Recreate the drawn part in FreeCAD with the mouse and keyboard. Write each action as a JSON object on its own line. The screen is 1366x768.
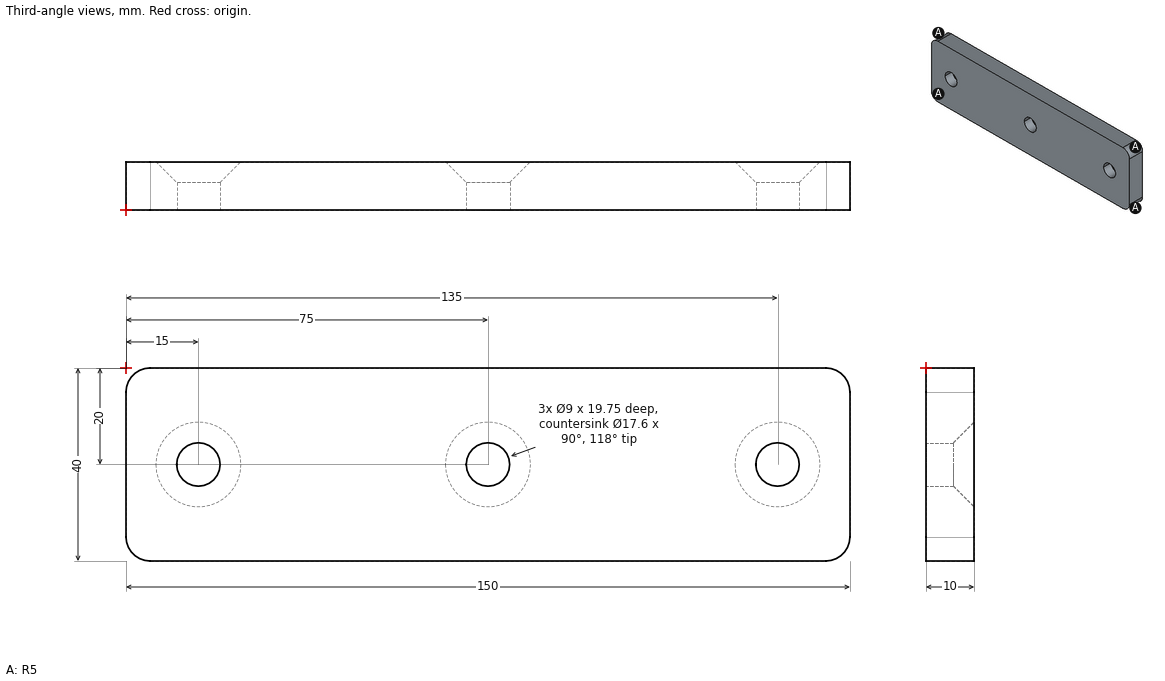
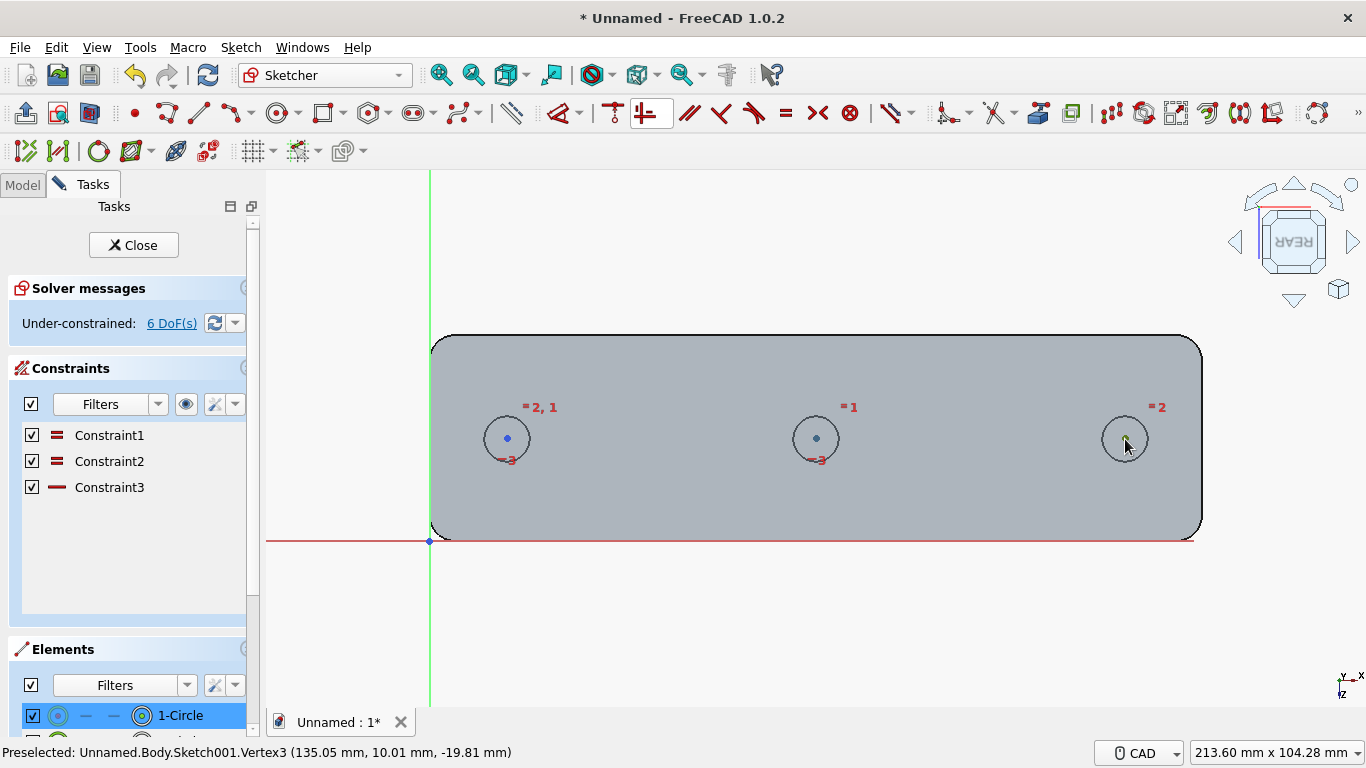
{"action": "left_click", "coordinate": [668, 114]}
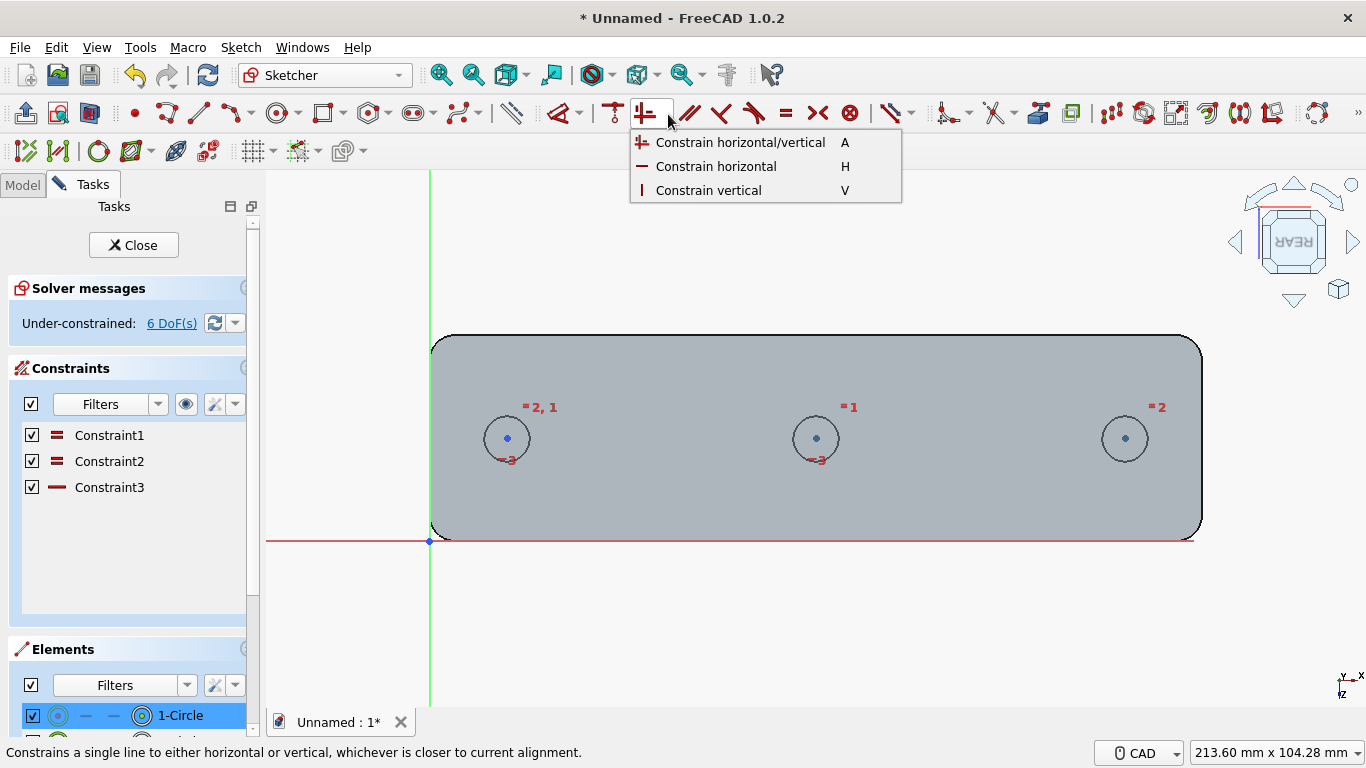
{"action": "left_click", "coordinate": [766, 166]}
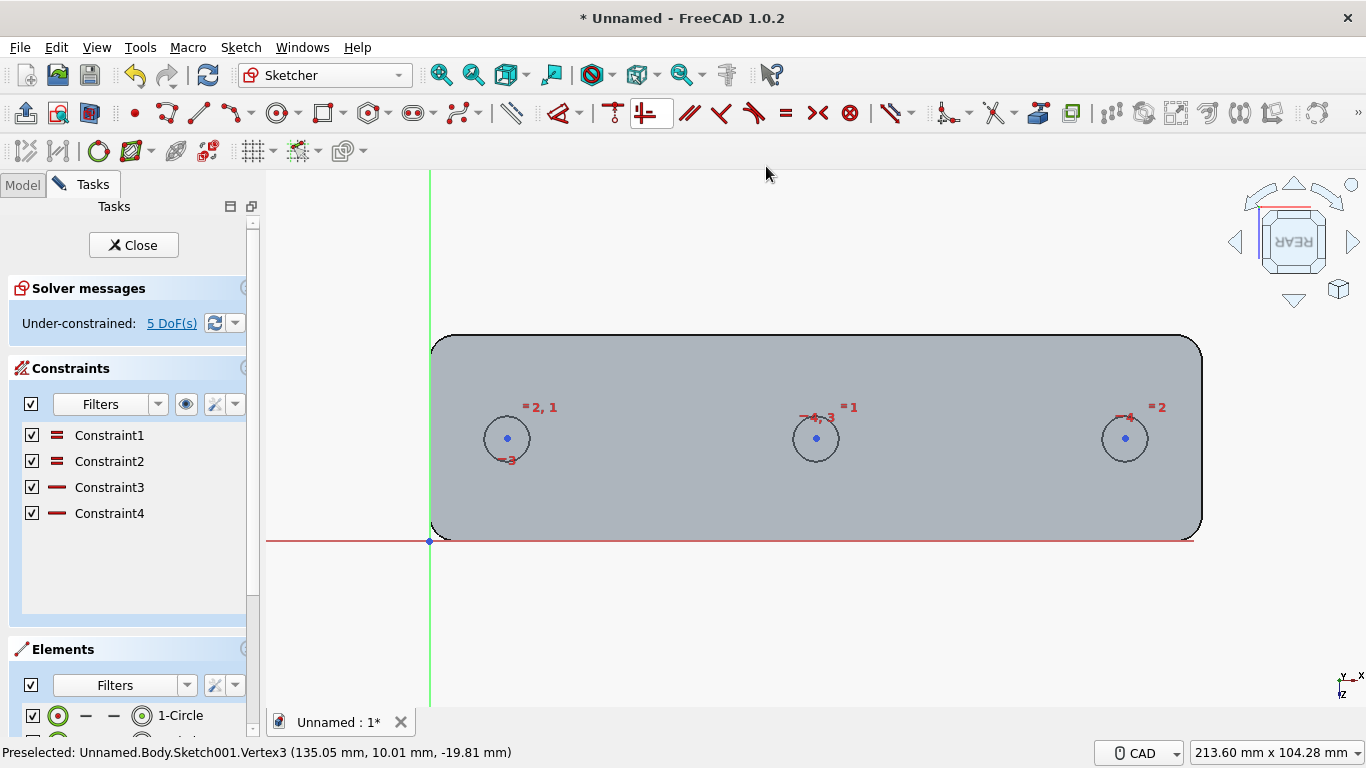
{"action": "left_click", "coordinate": [558, 114]}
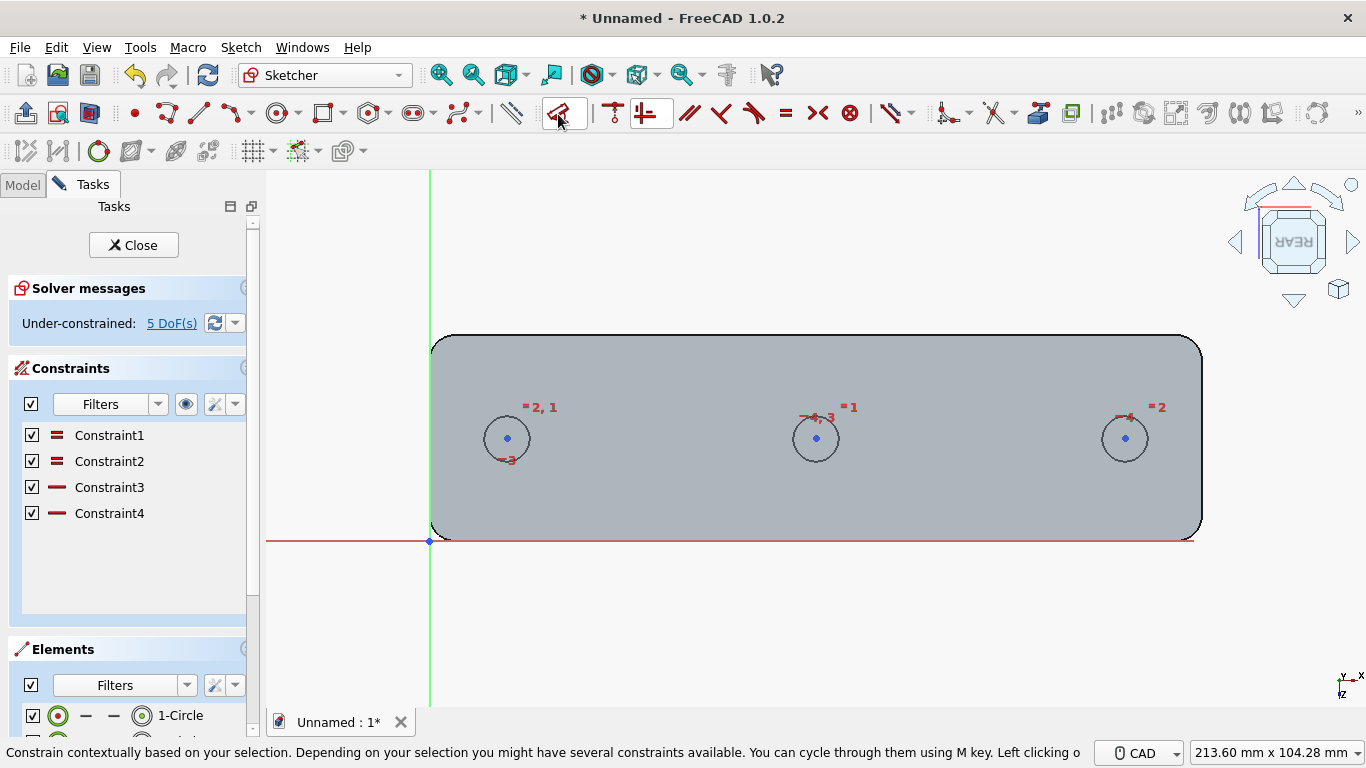
{"action": "left_click", "coordinate": [832, 423]}
{"action": "left_click", "coordinate": [855, 400]}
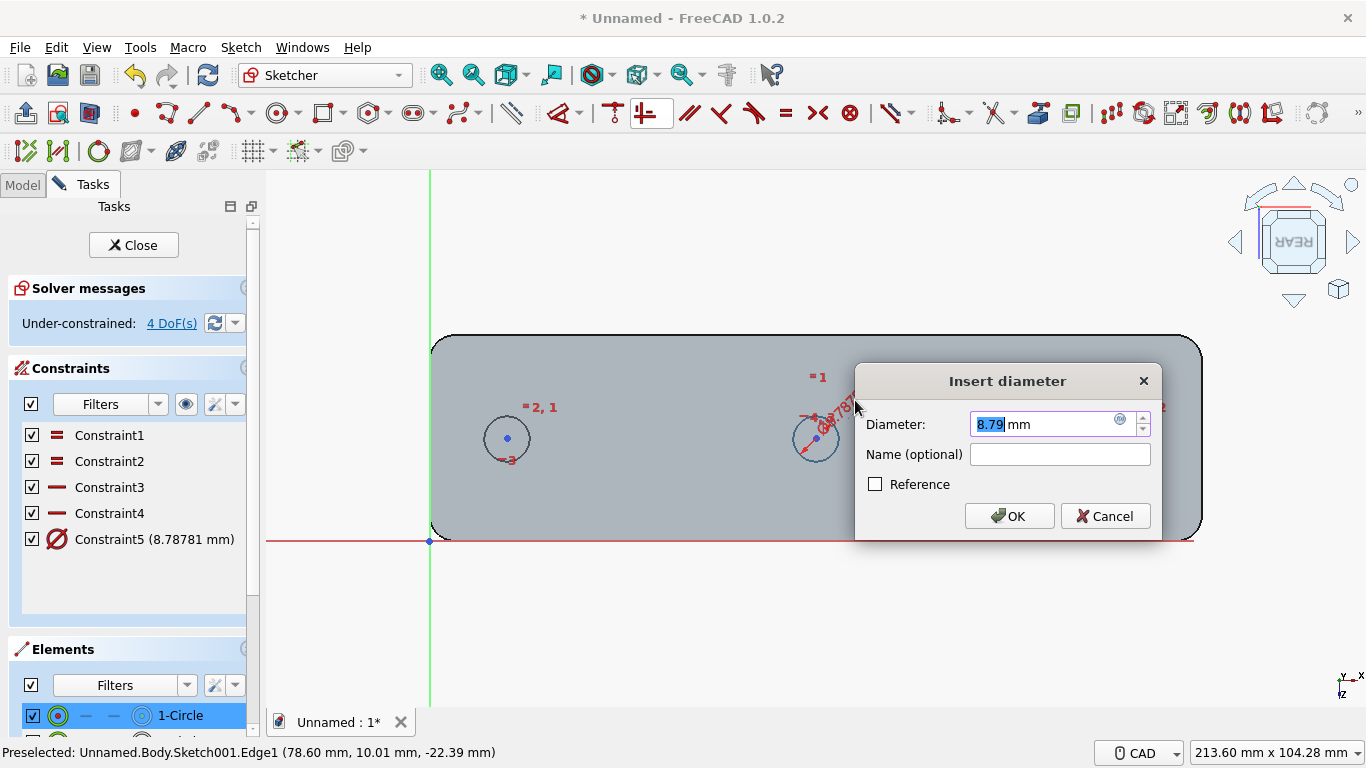
{"action": "type", "text": "9"}
{"action": "key", "text": "Return"}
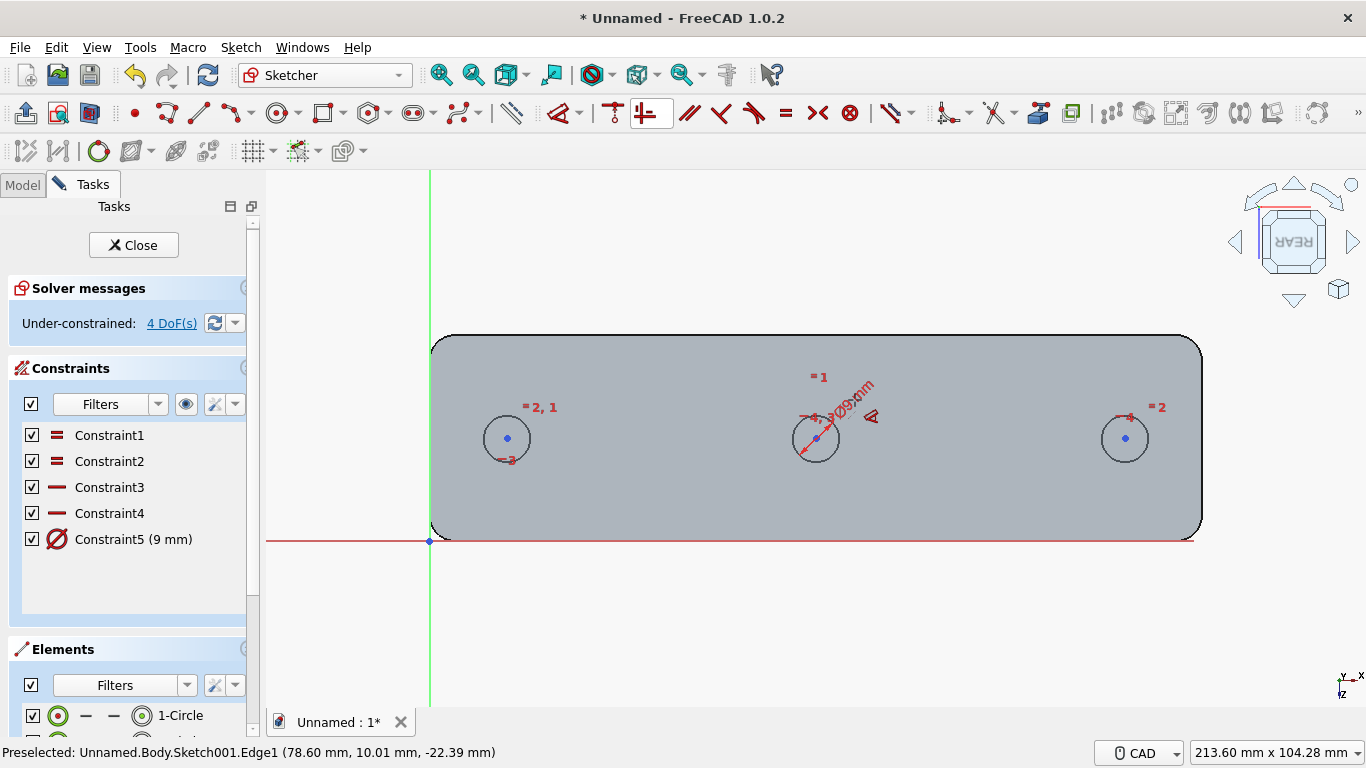
{"action": "left_click", "coordinate": [816, 439]}
{"action": "left_click", "coordinate": [623, 575]}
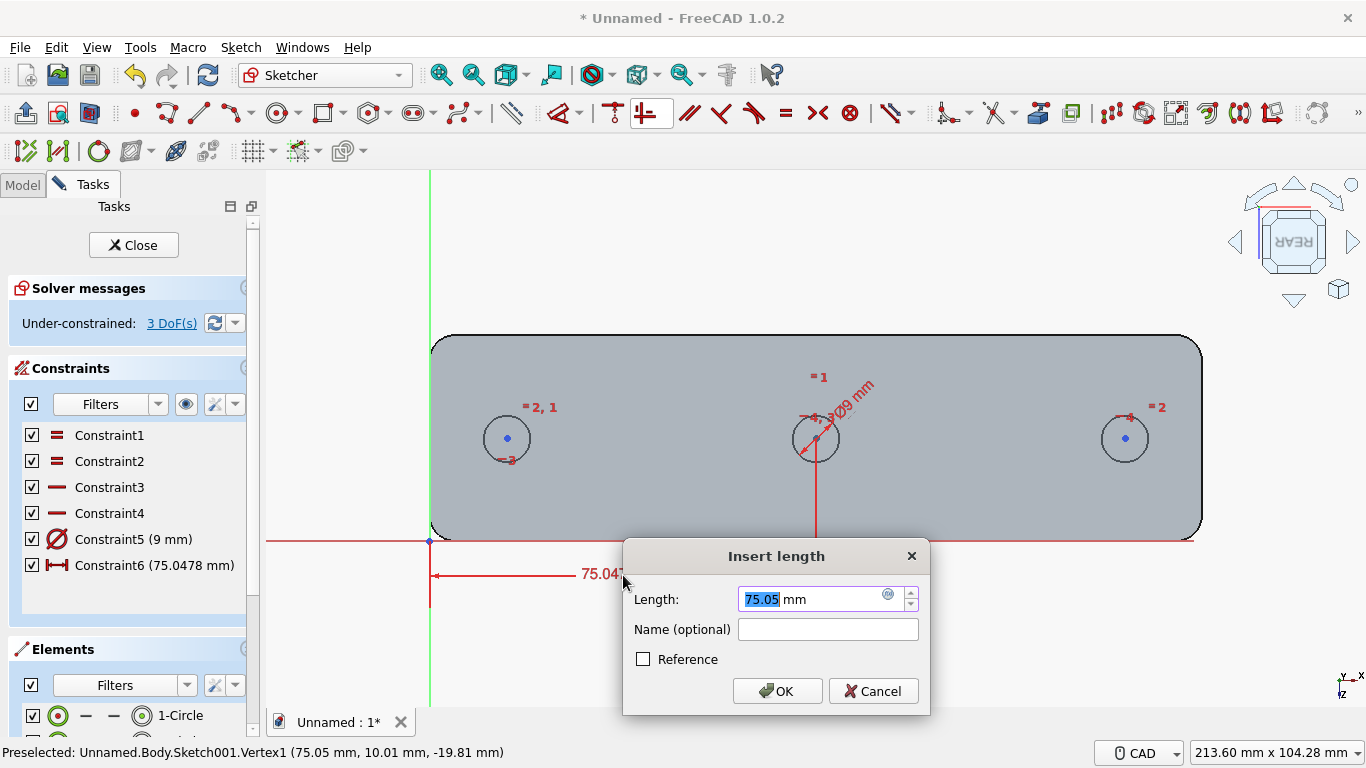
{"action": "type", "text": "75"}
{"action": "key", "text": "Return"}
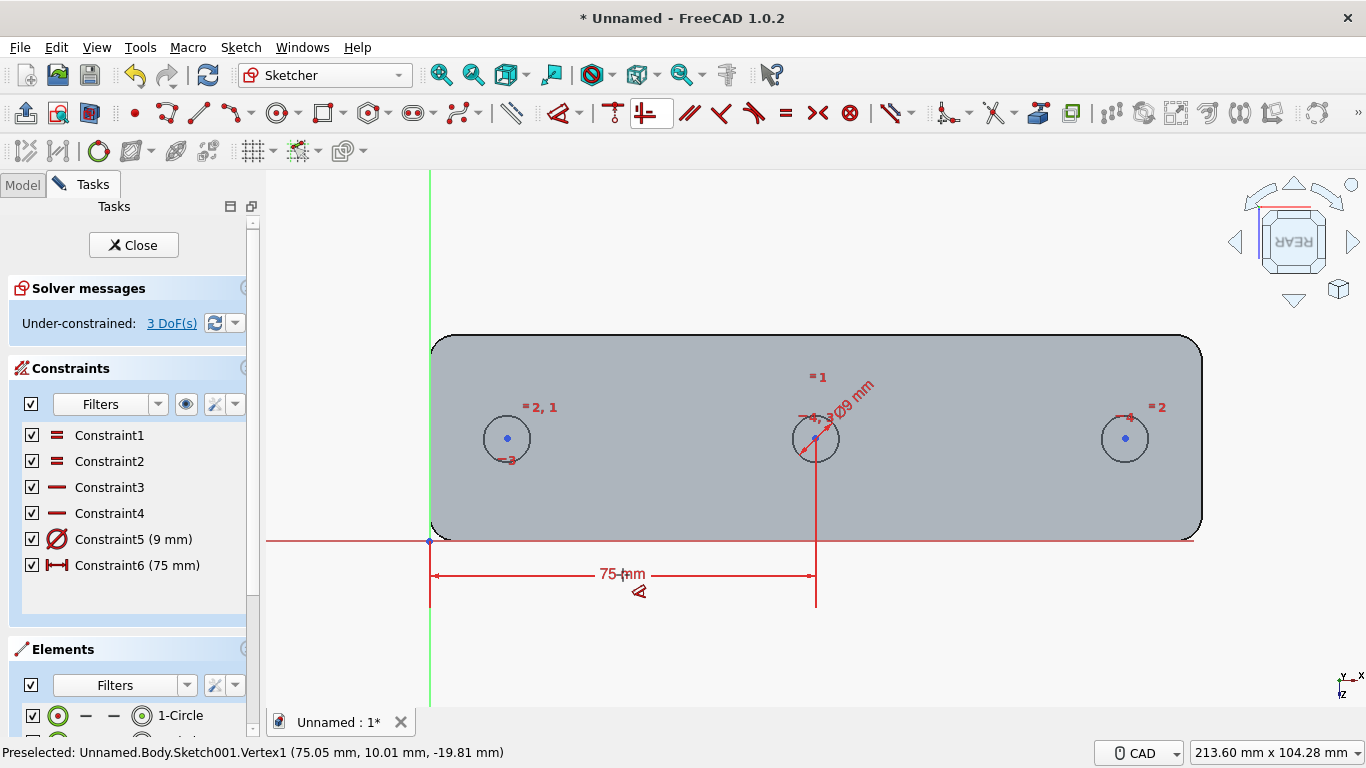
{"action": "left_click", "coordinate": [816, 439]}
{"action": "left_click", "coordinate": [396, 490]}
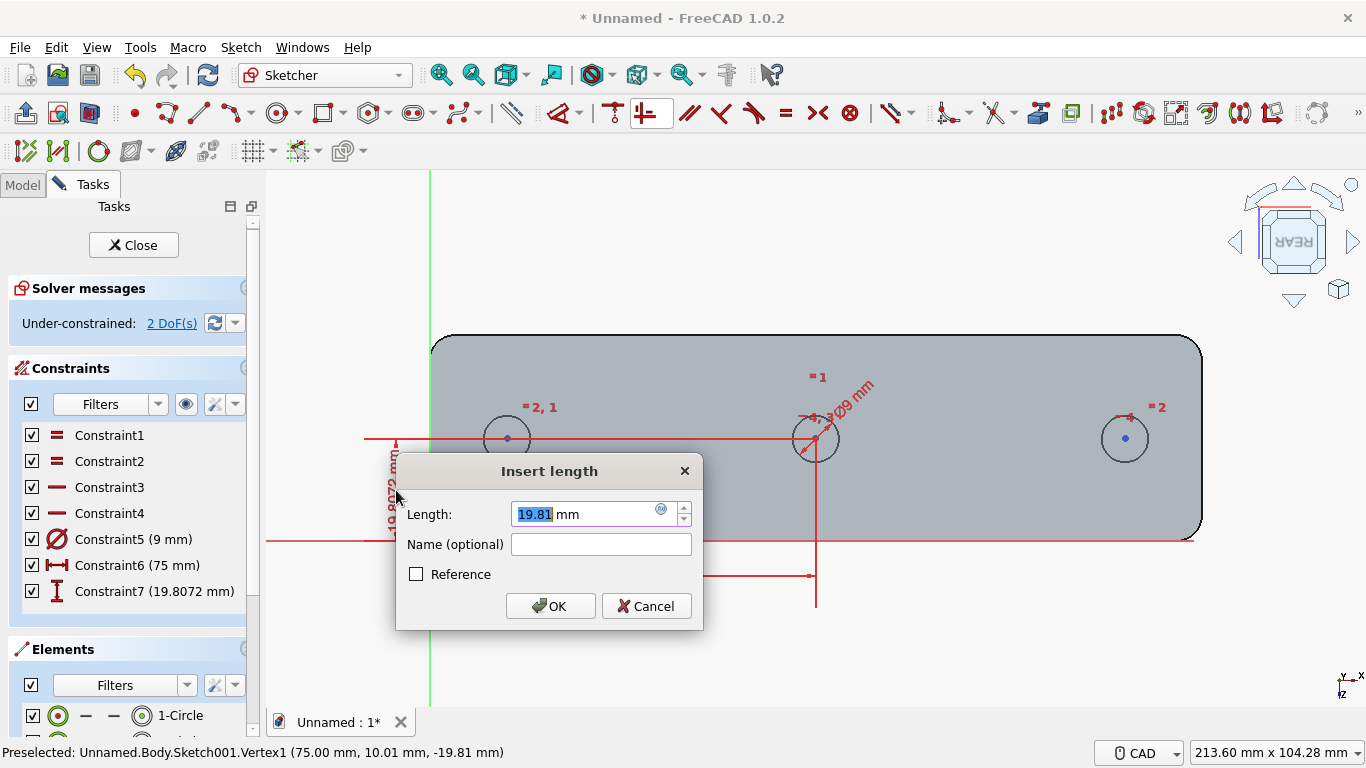
{"action": "type", "text": "20"}
{"action": "key", "text": "Return"}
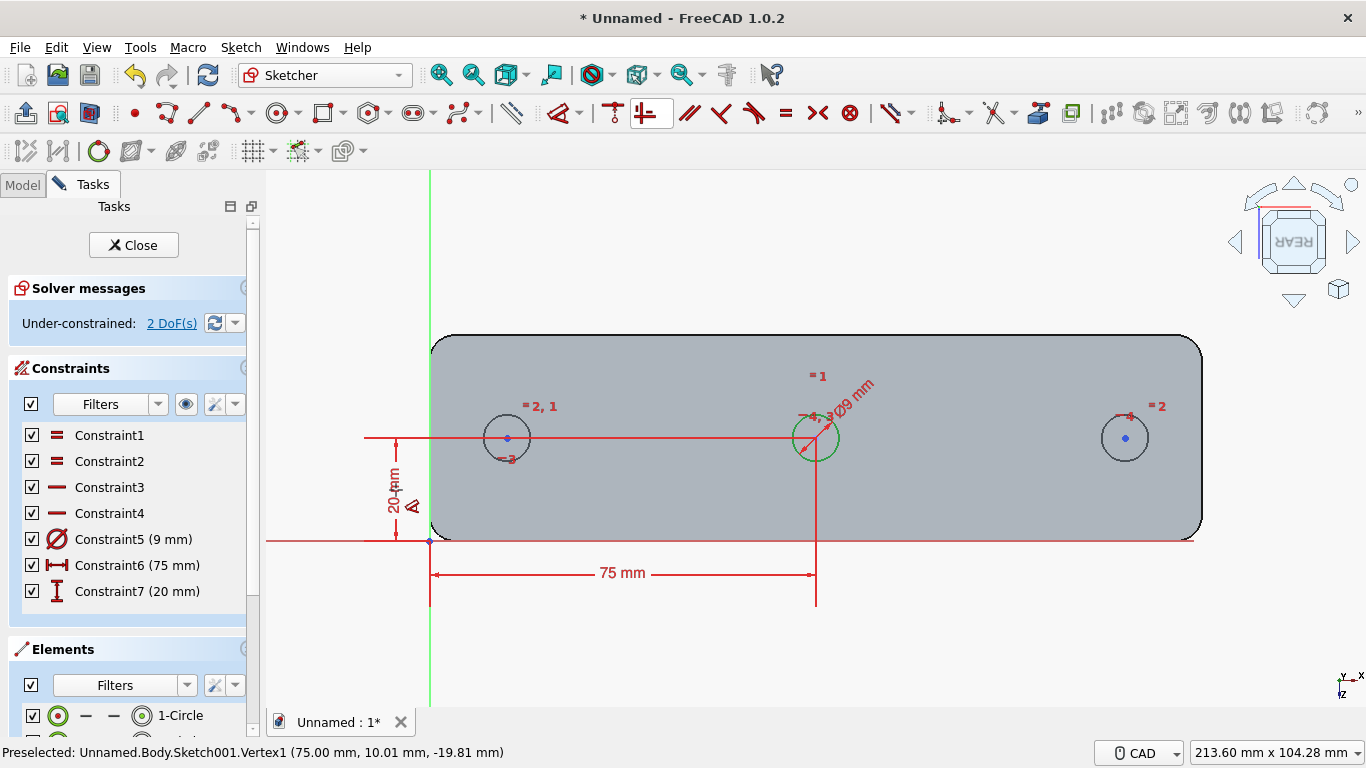
{"action": "left_click", "coordinate": [507, 438]}
{"action": "left_click", "coordinate": [468, 575]}